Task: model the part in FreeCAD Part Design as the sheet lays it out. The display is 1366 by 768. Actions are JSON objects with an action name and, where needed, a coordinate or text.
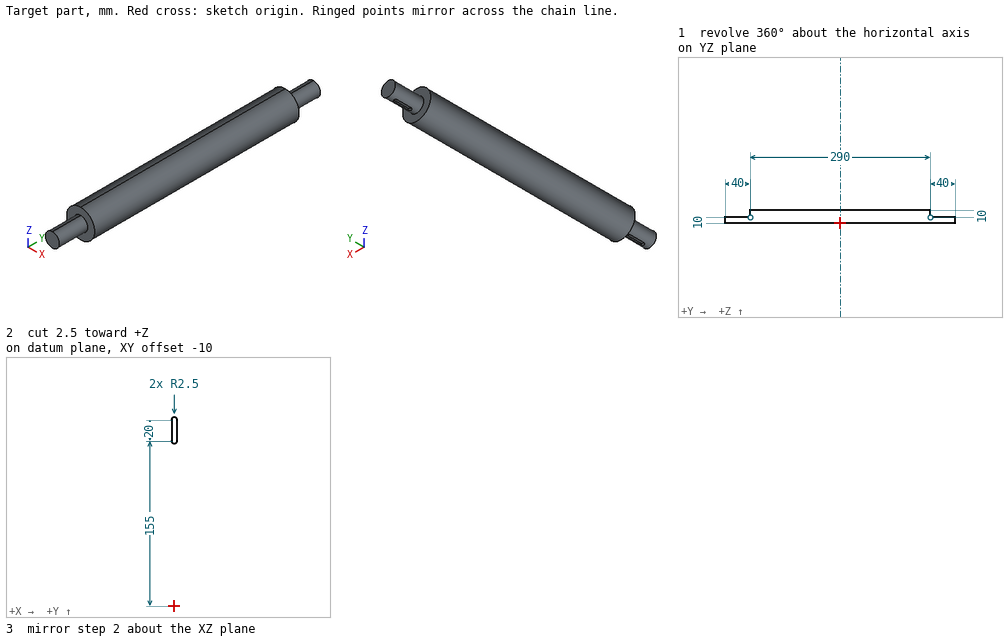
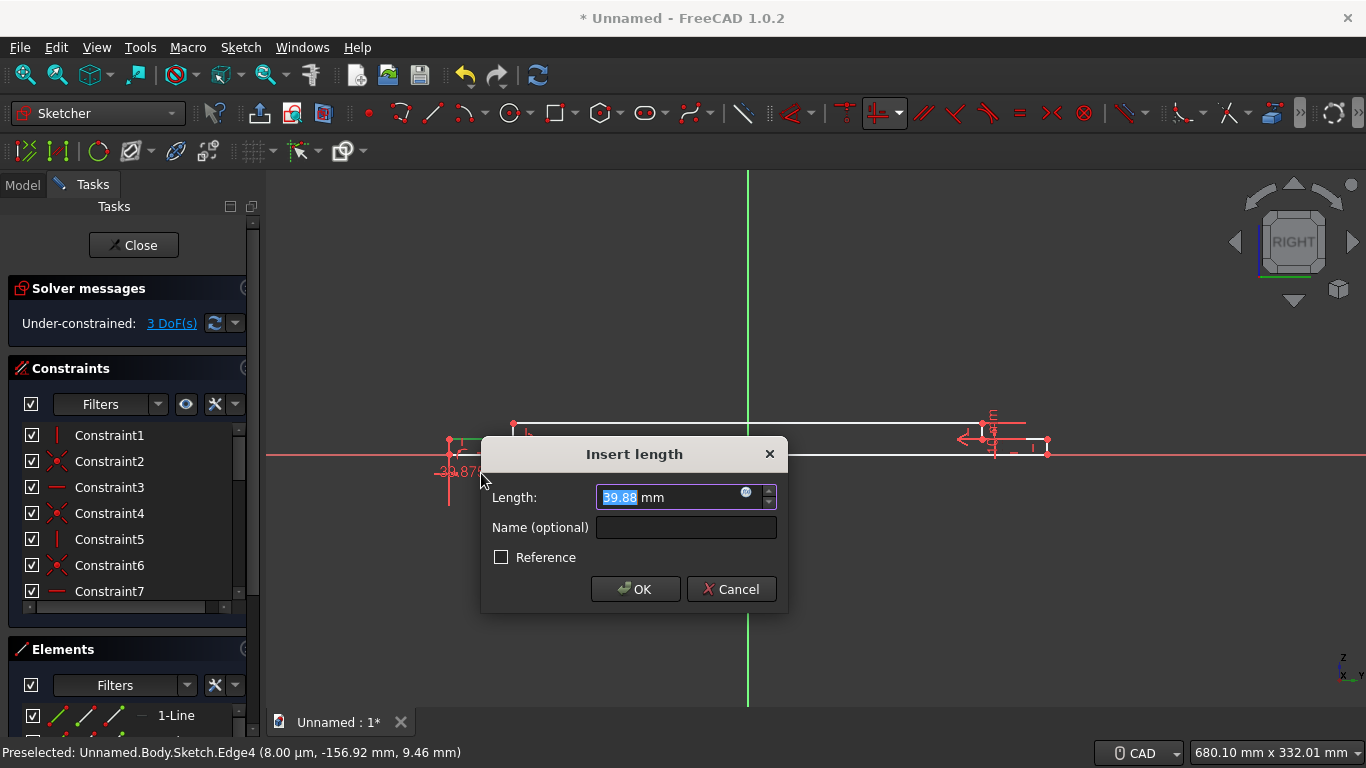
{"action": "type", "text": "40"}
{"action": "key", "text": "Return"}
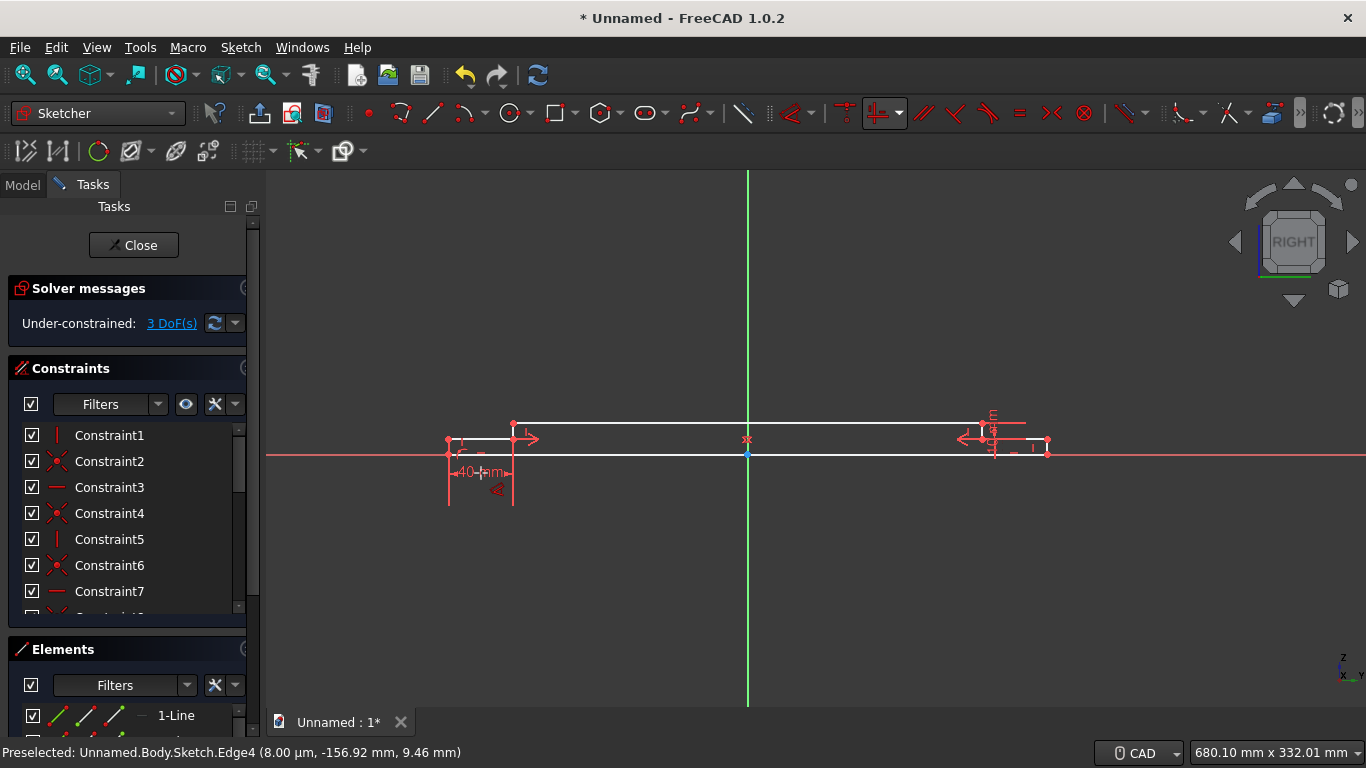
{"action": "scroll", "coordinate": [449, 447], "scroll_direction": "up", "scroll_amount": 5}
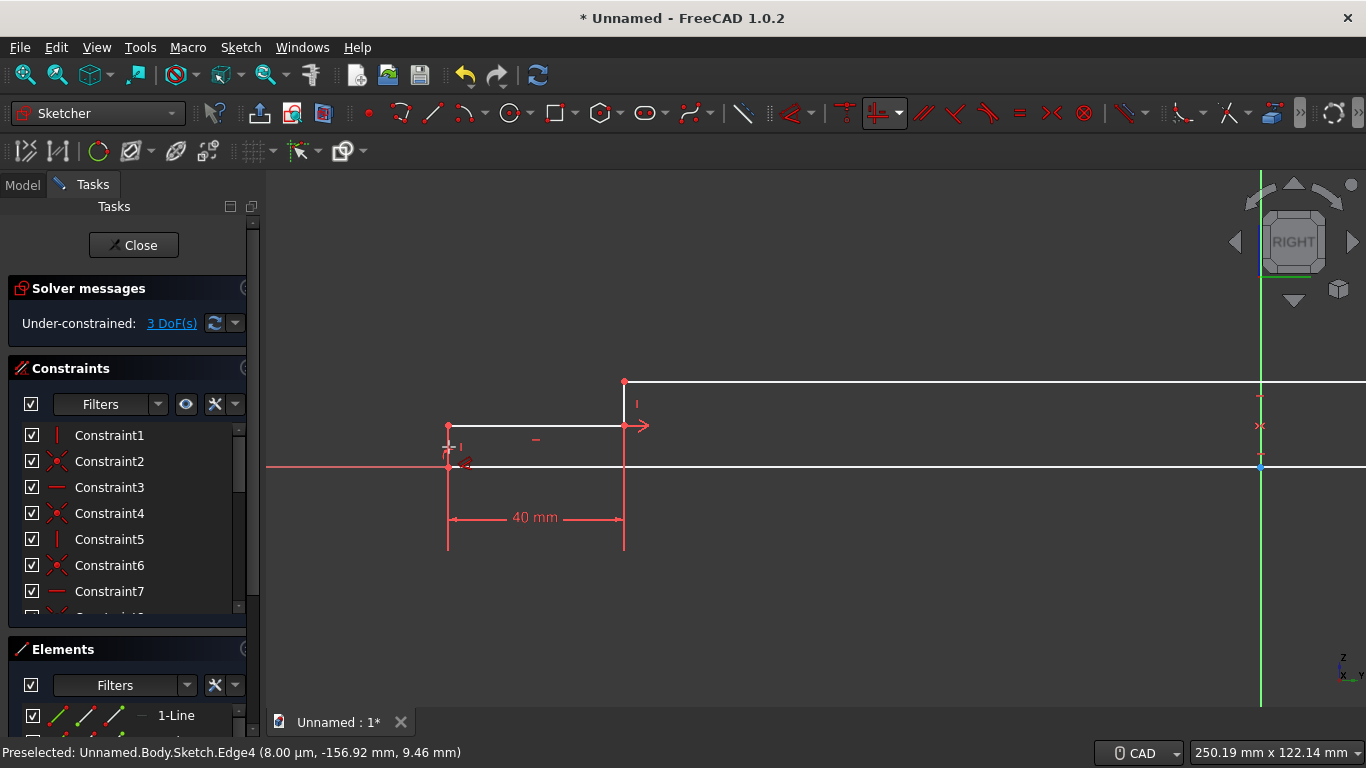
{"action": "left_click", "coordinate": [448, 446]}
{"action": "left_click", "coordinate": [414, 446]}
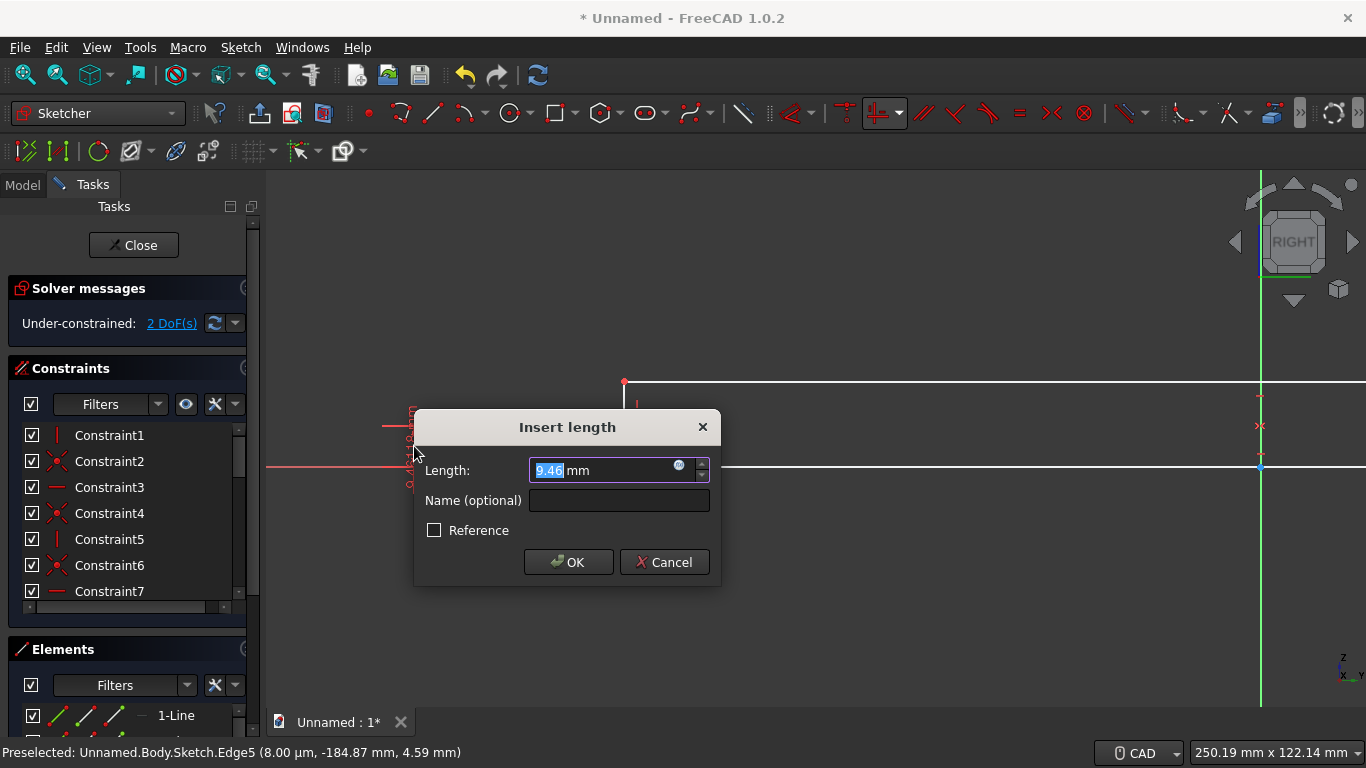
{"action": "type", "text": "10"}
{"action": "key", "text": "Return"}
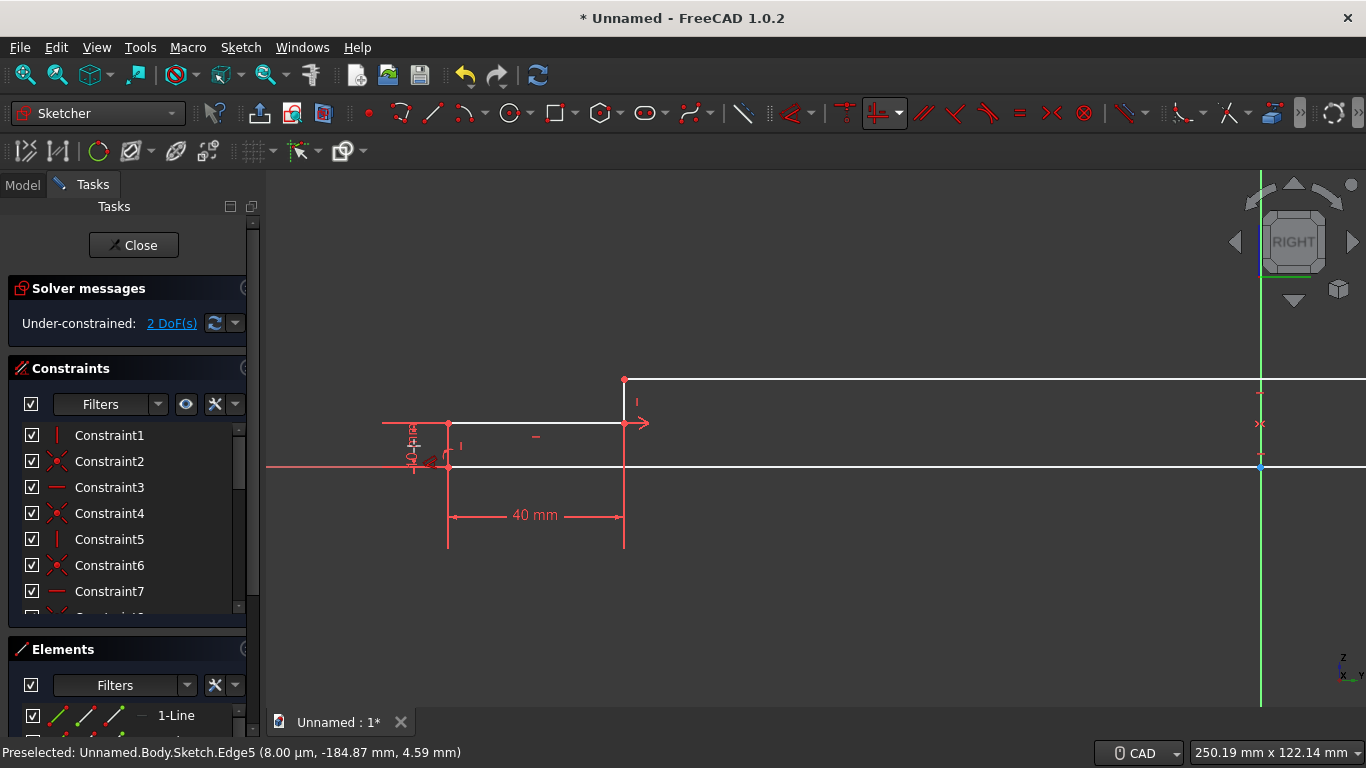
{"action": "scroll", "coordinate": [449, 447], "scroll_direction": "down", "scroll_amount": 5}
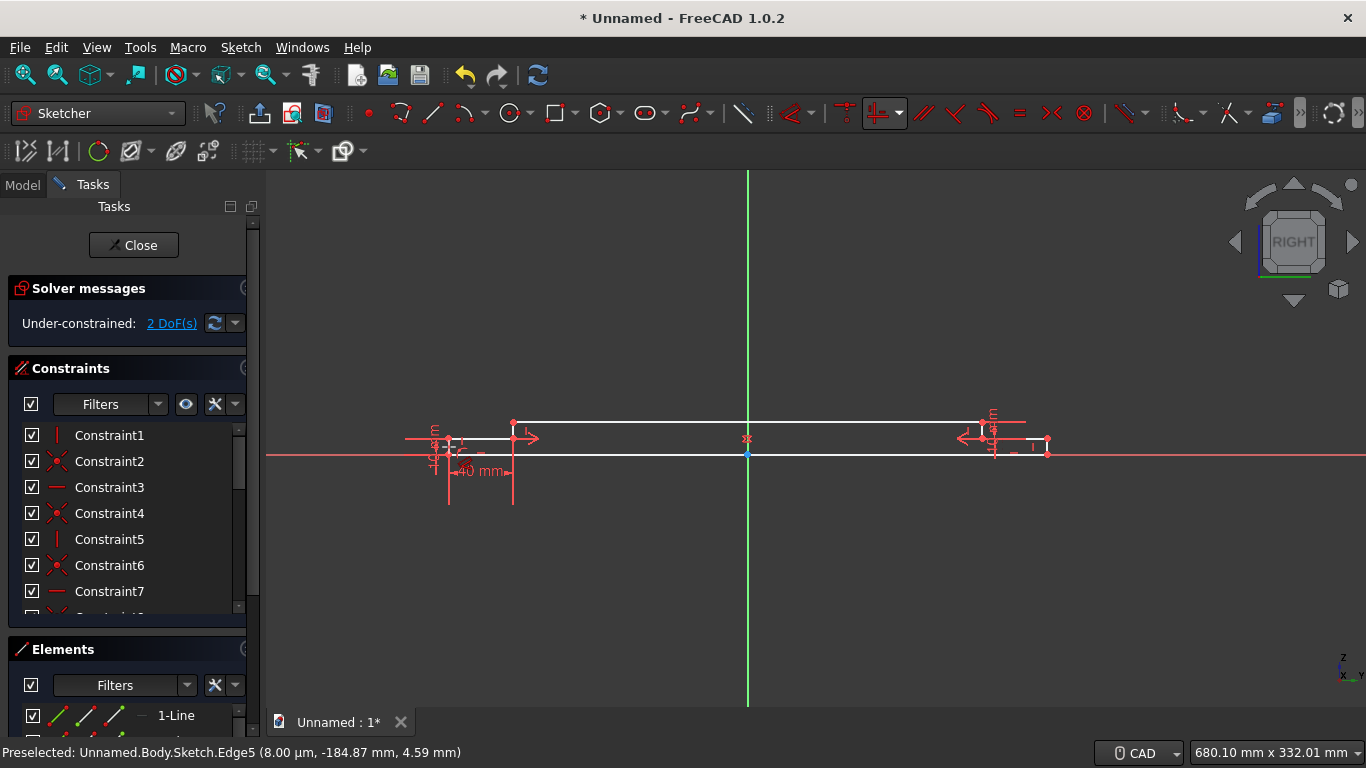
{"action": "left_click", "coordinate": [1028, 439]}
{"action": "left_click", "coordinate": [1015, 473]}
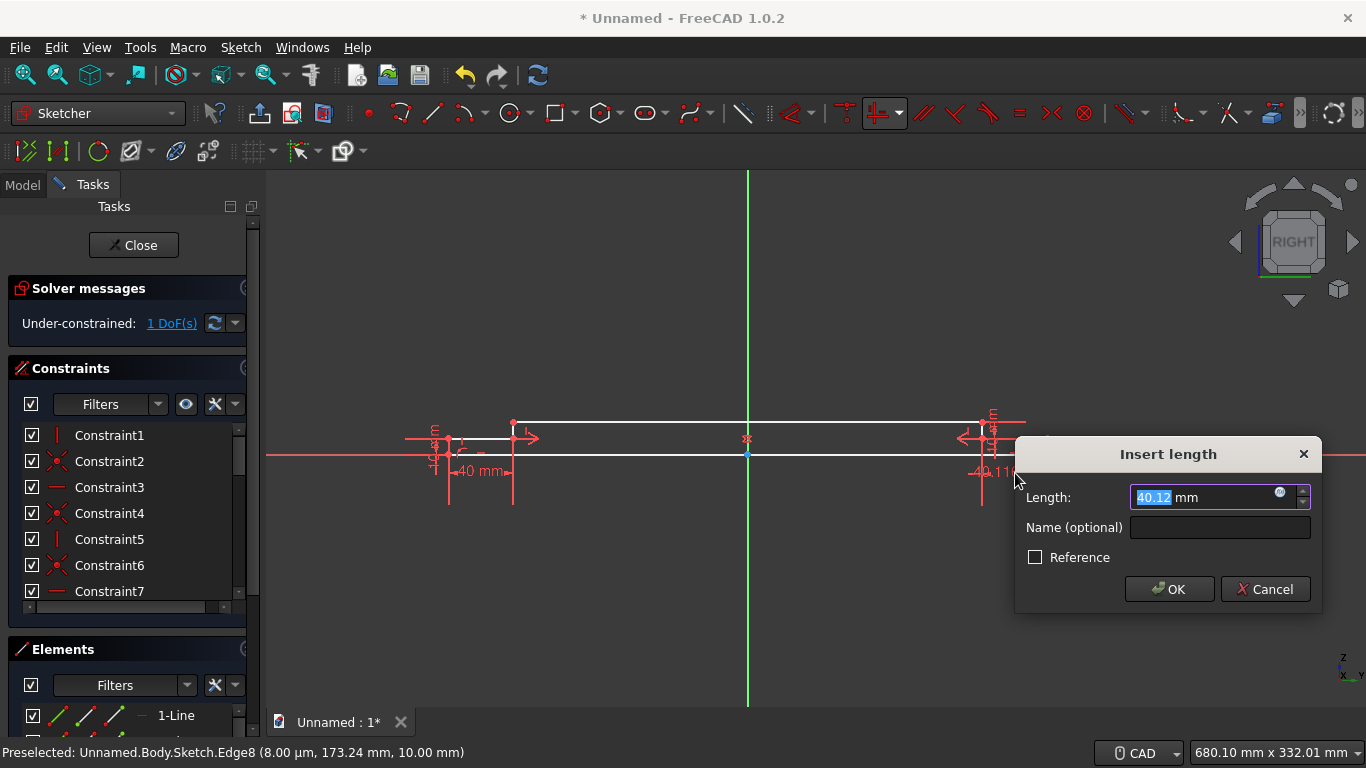
{"action": "type", "text": "40"}
{"action": "key", "text": "Return"}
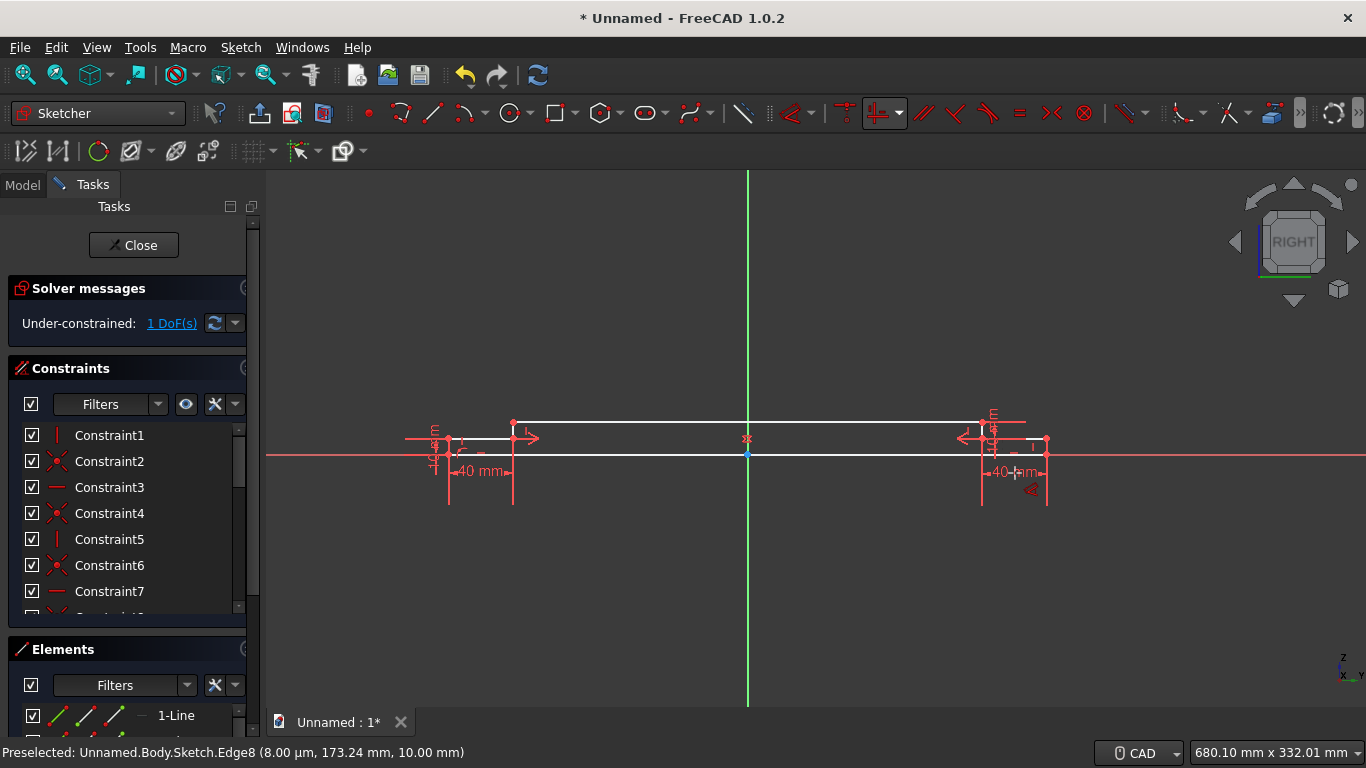
{"action": "left_click", "coordinate": [842, 422]}
{"action": "left_click", "coordinate": [640, 388]}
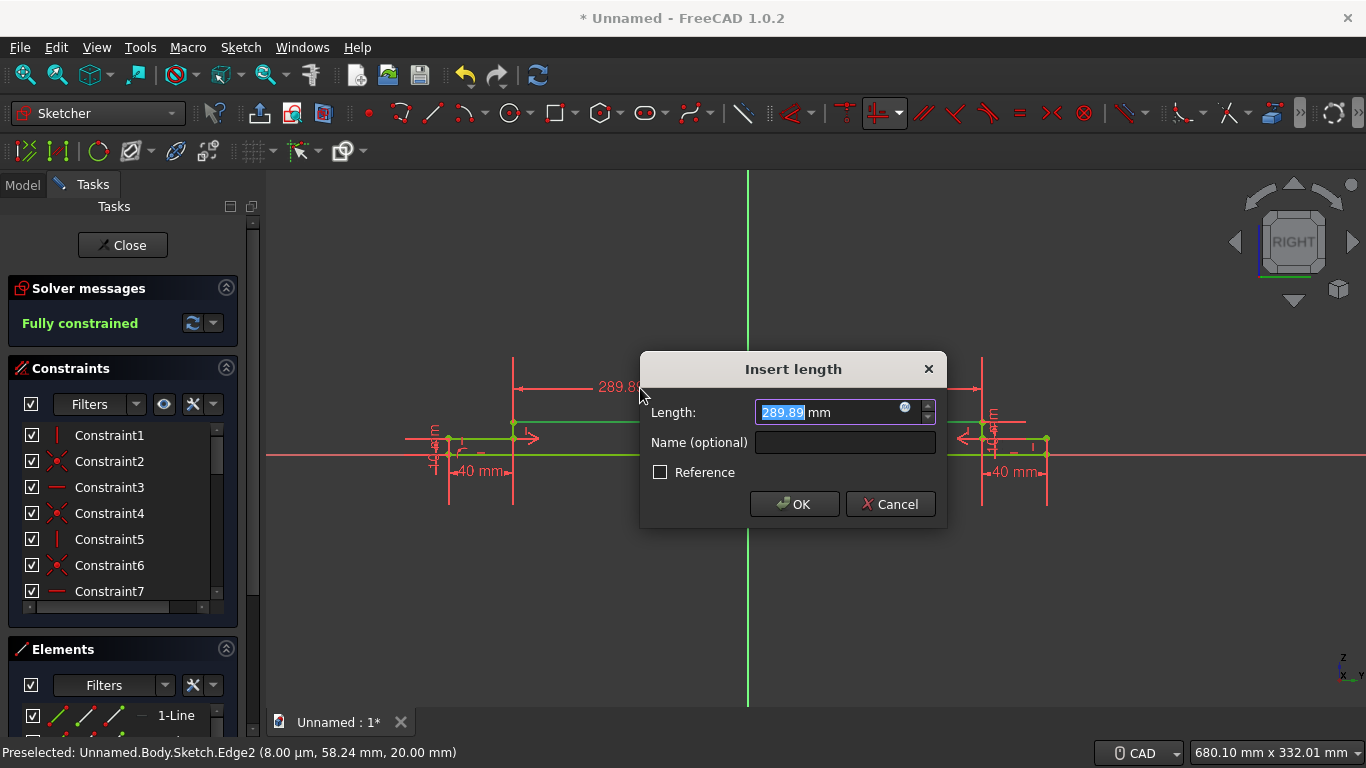
{"action": "type", "text": "290"}
{"action": "key", "text": "Return"}
{"action": "key", "text": "Escape"}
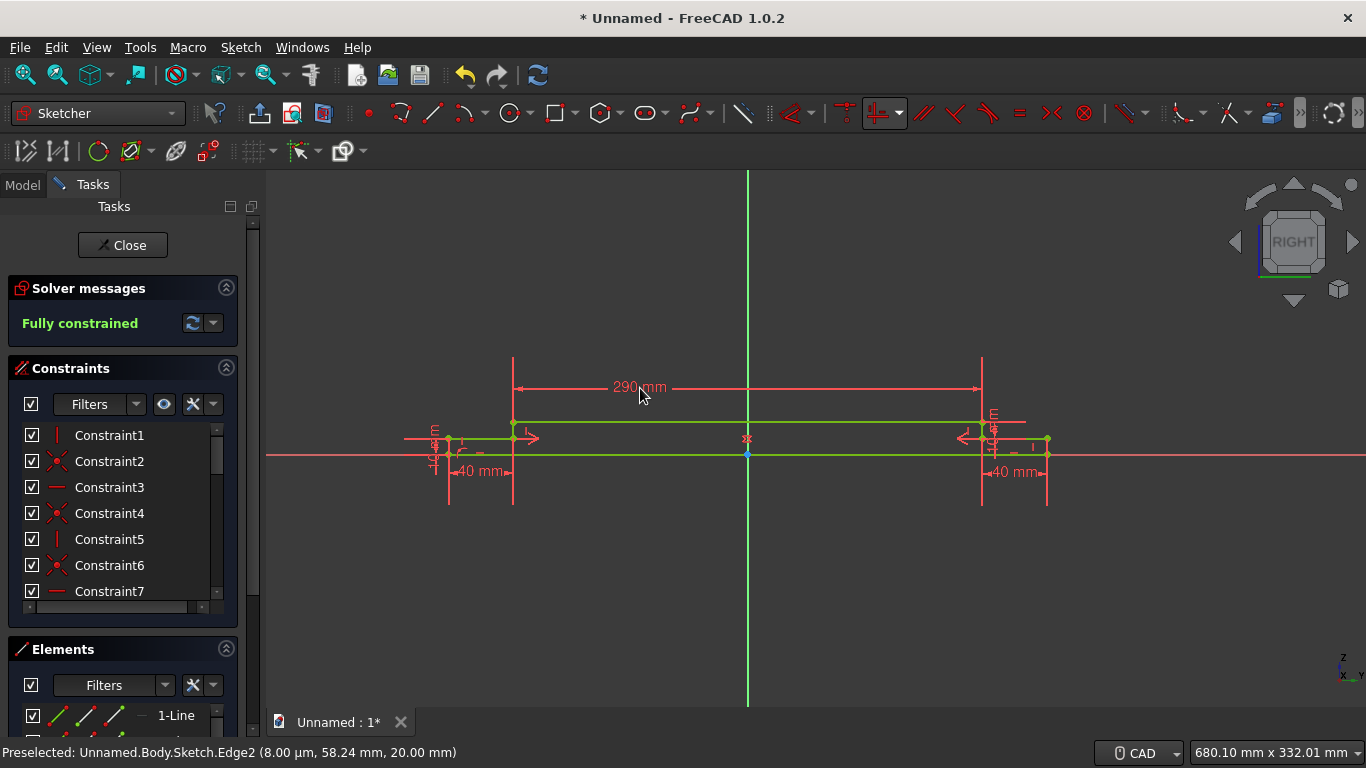
{"action": "left_click", "coordinate": [123, 245]}